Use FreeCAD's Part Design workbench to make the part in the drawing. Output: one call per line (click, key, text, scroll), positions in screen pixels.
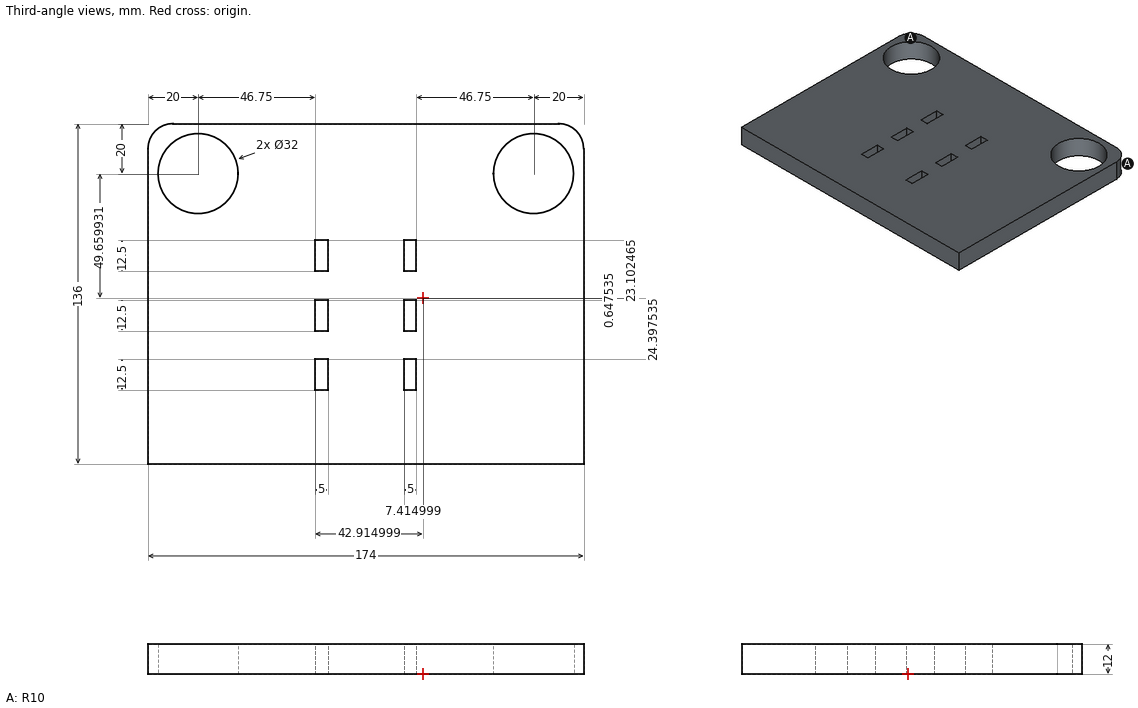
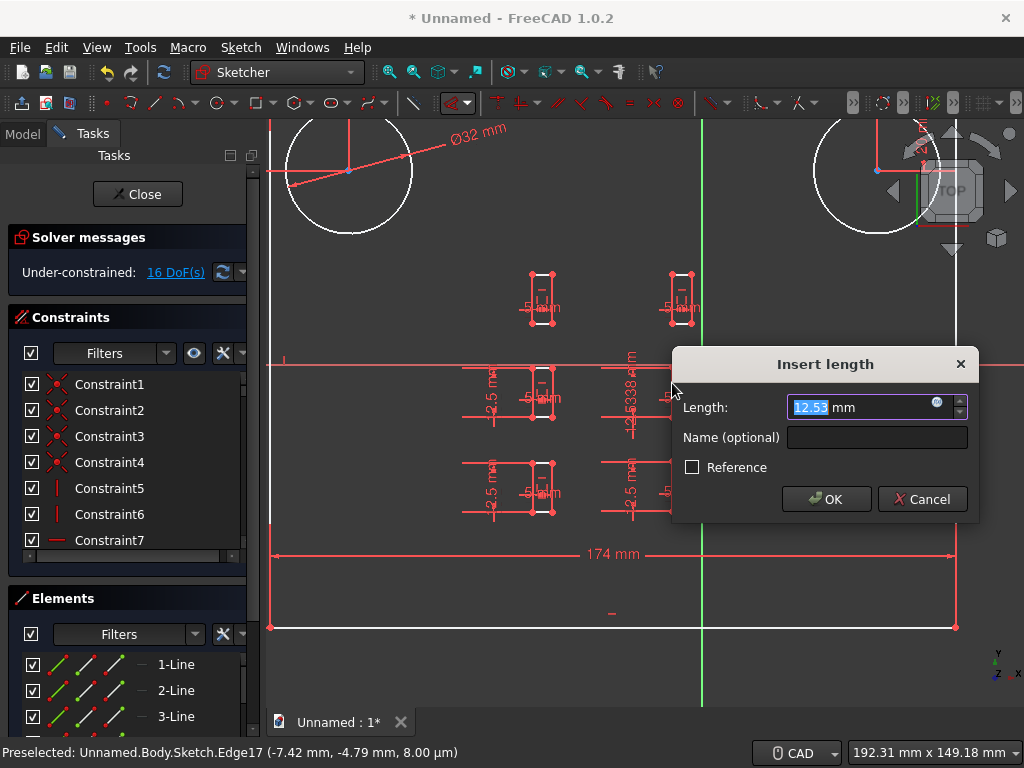
text(12.5)
key(Return)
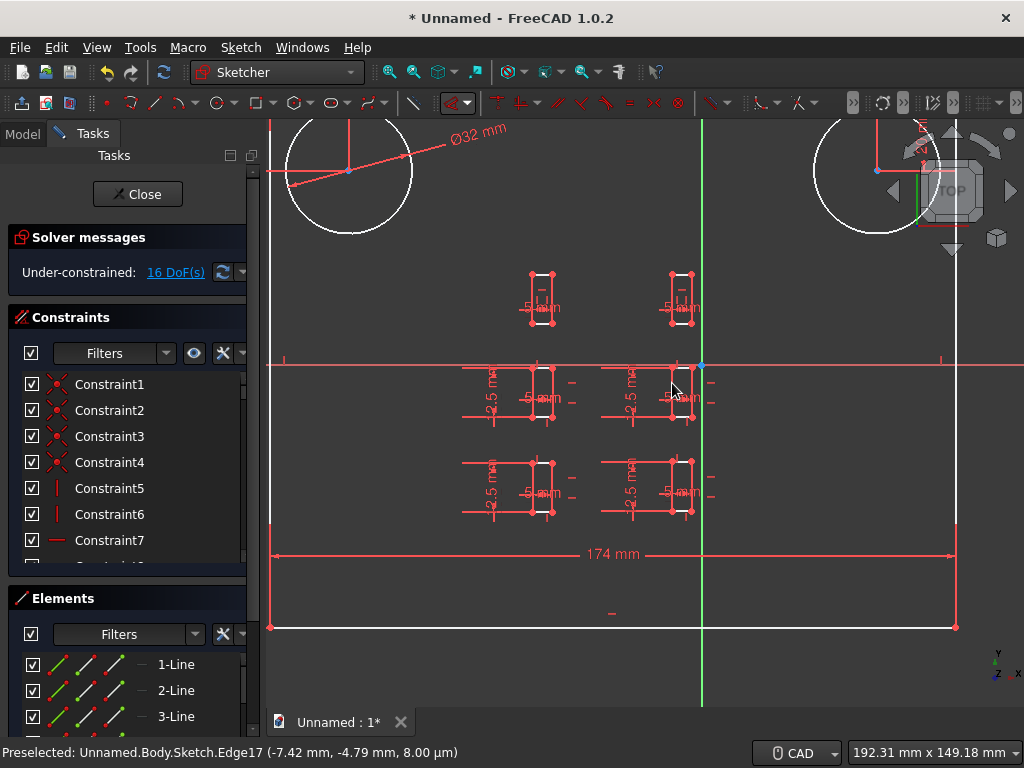
click(532, 289)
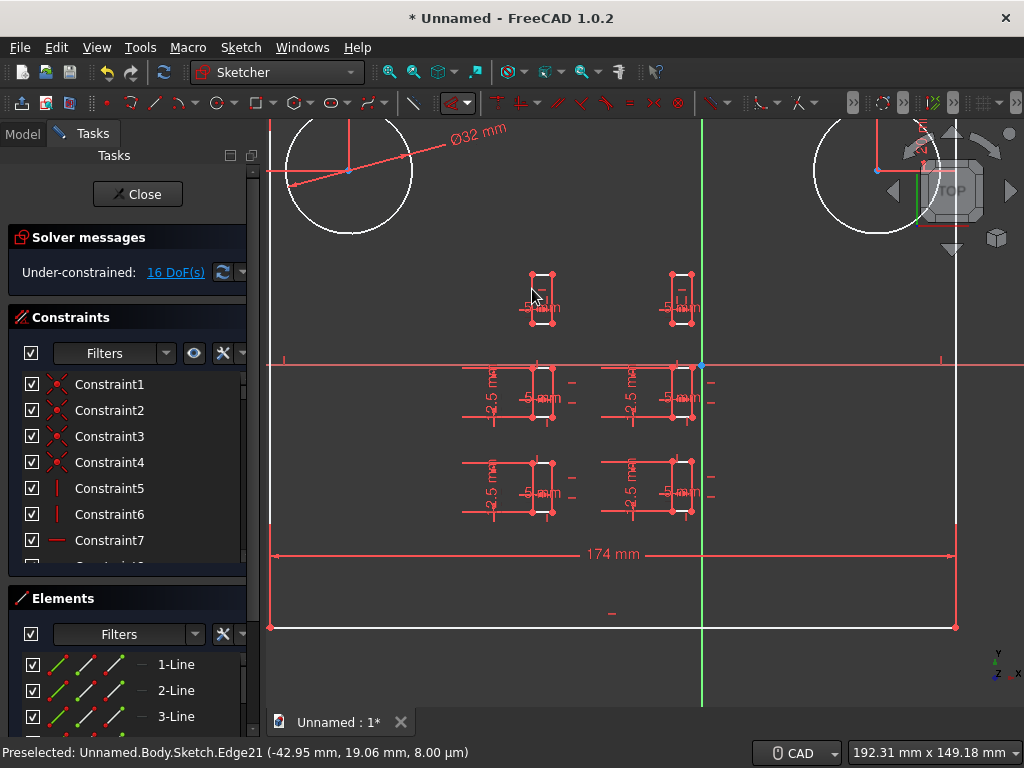
click(470, 104)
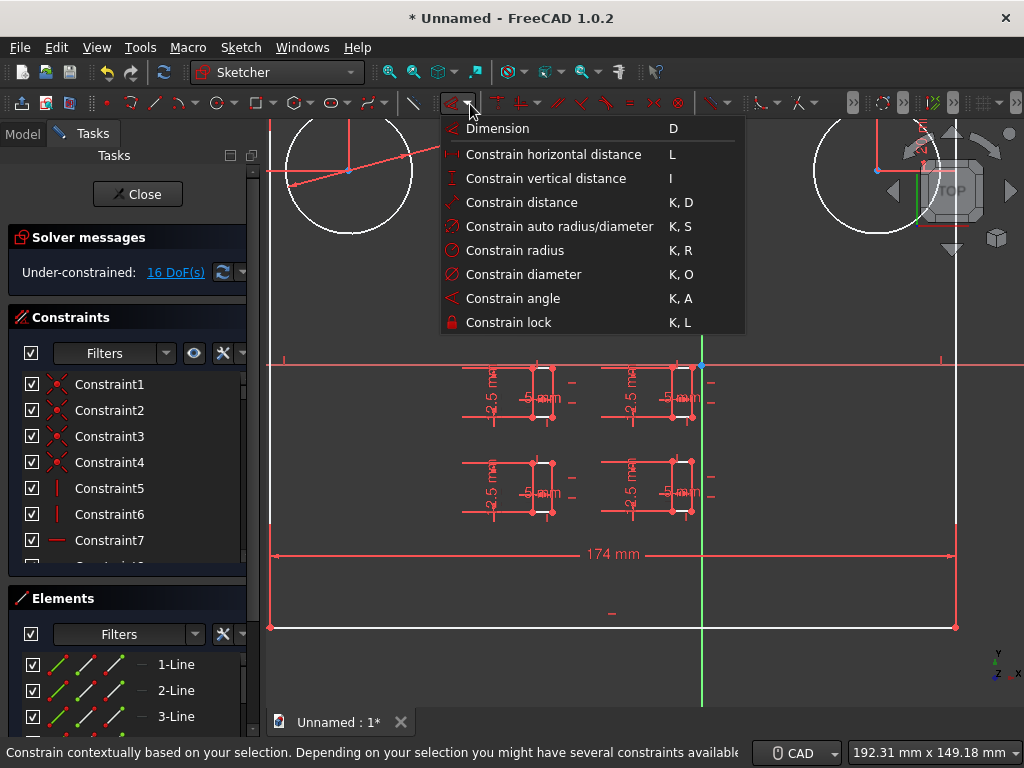
click(593, 178)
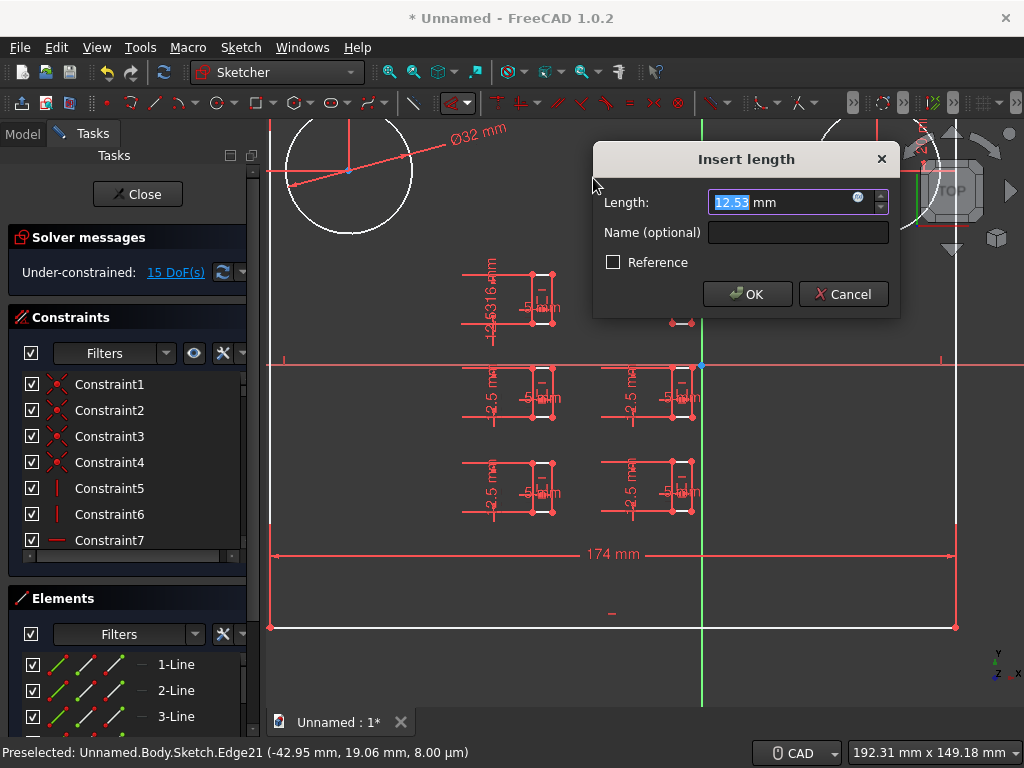
text(12.5)
key(Return)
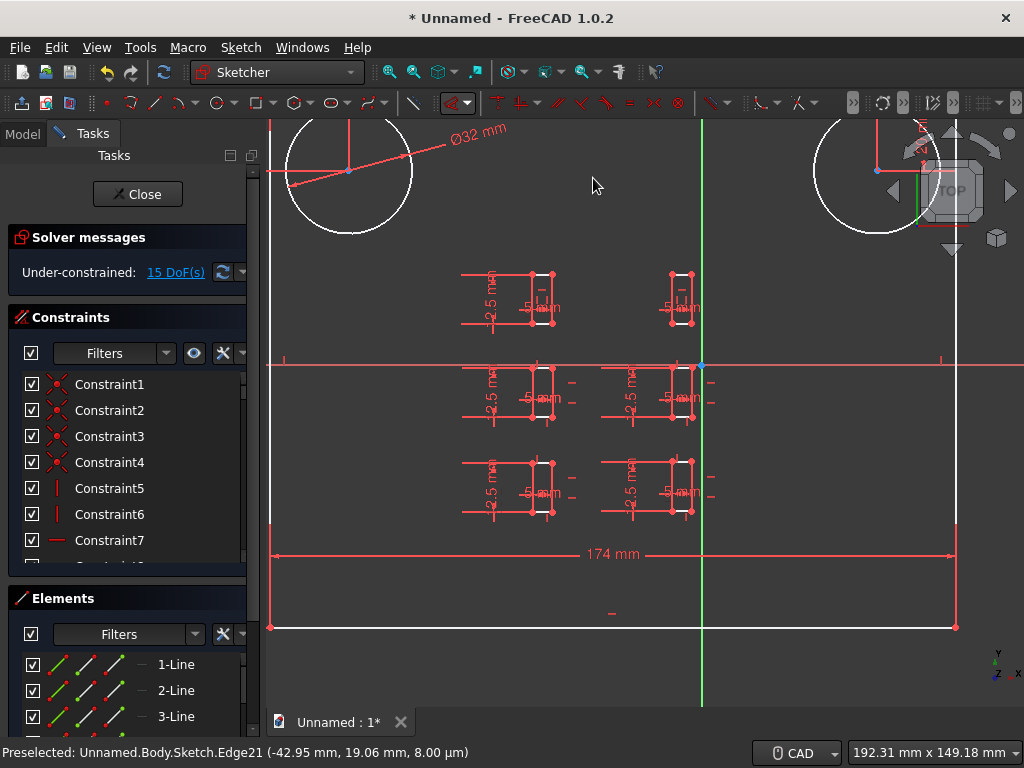
click(672, 289)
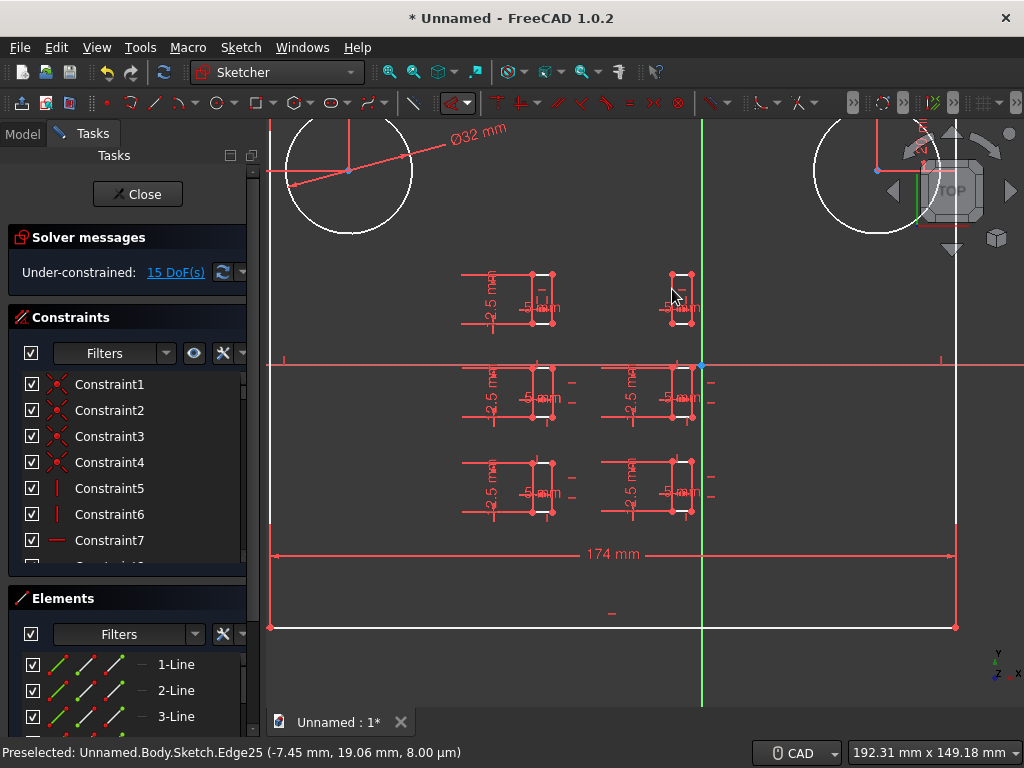
key(i)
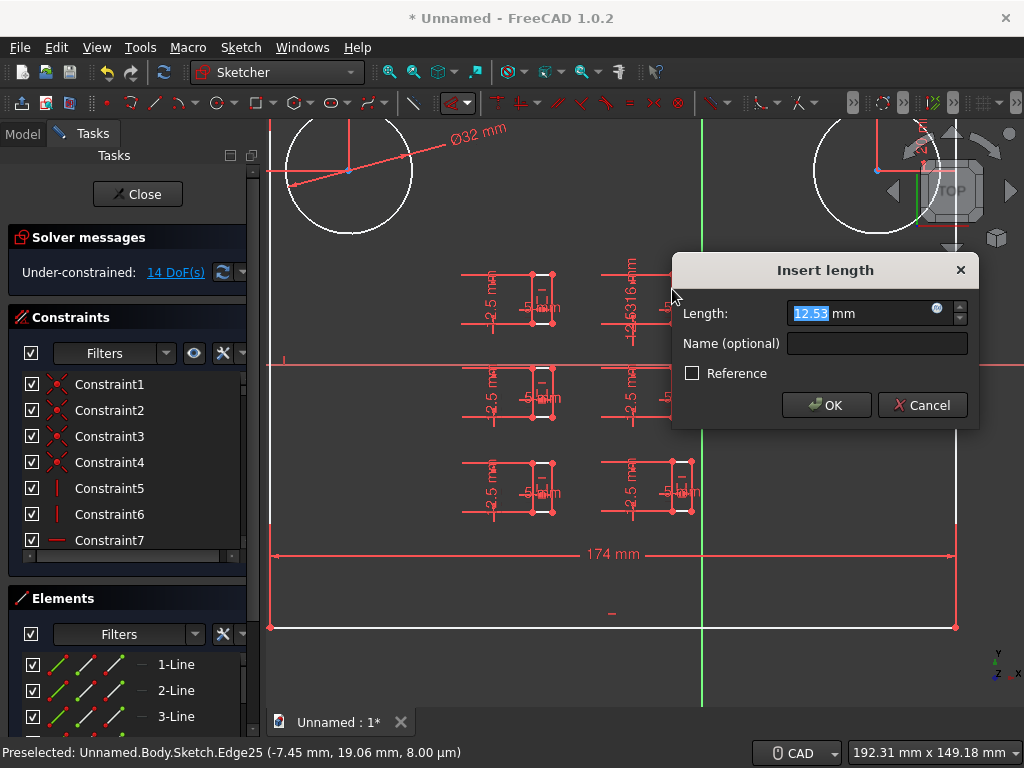
text(12.5)
key(Return)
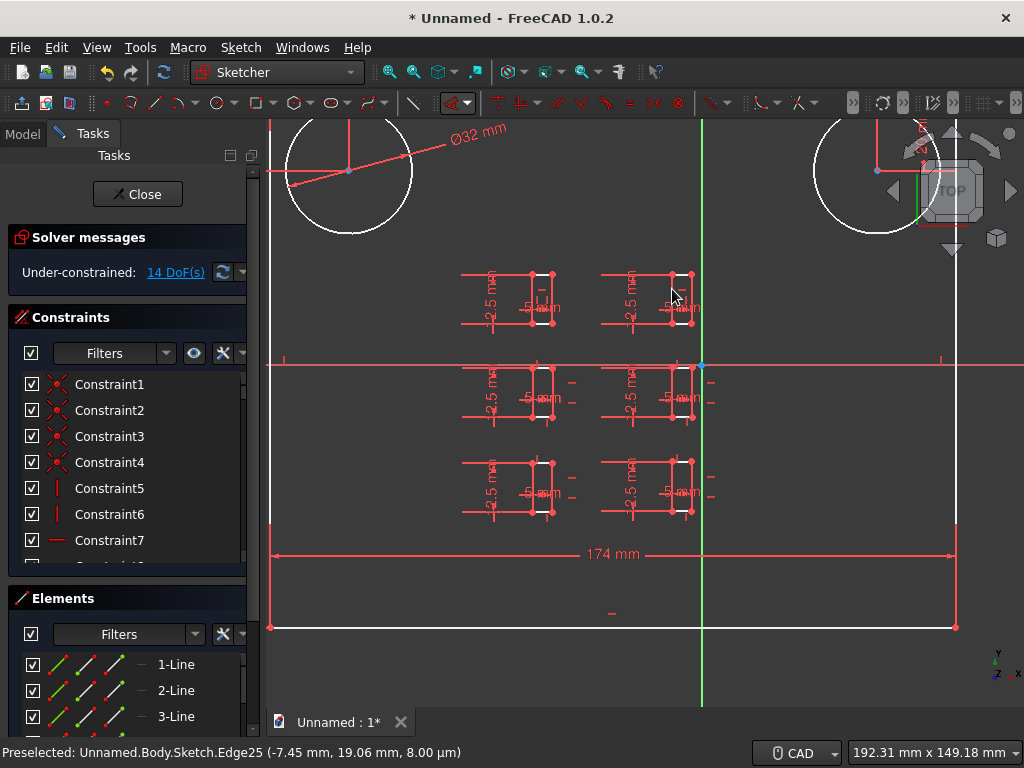
click(532, 275)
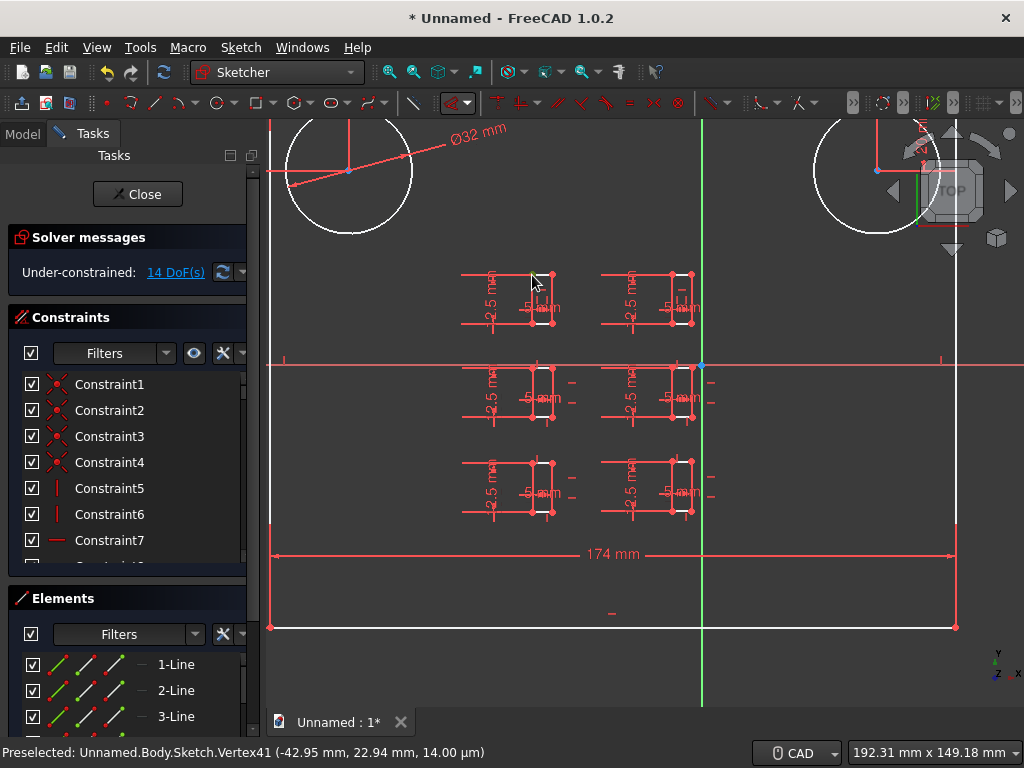
click(349, 171)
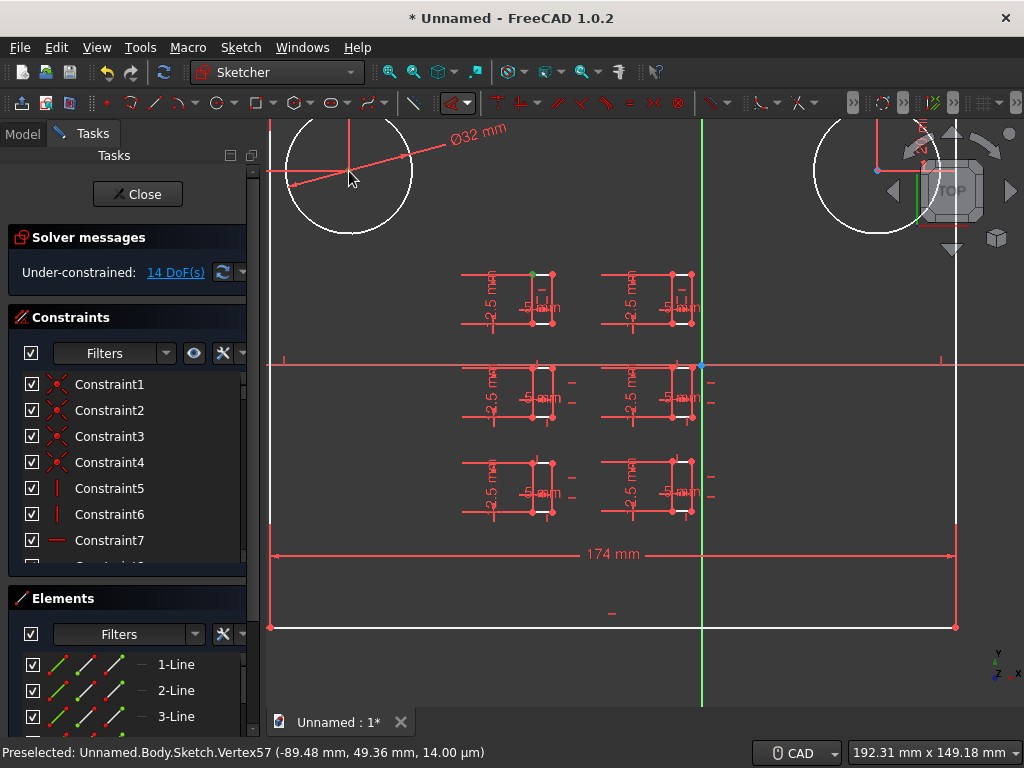
click(470, 104)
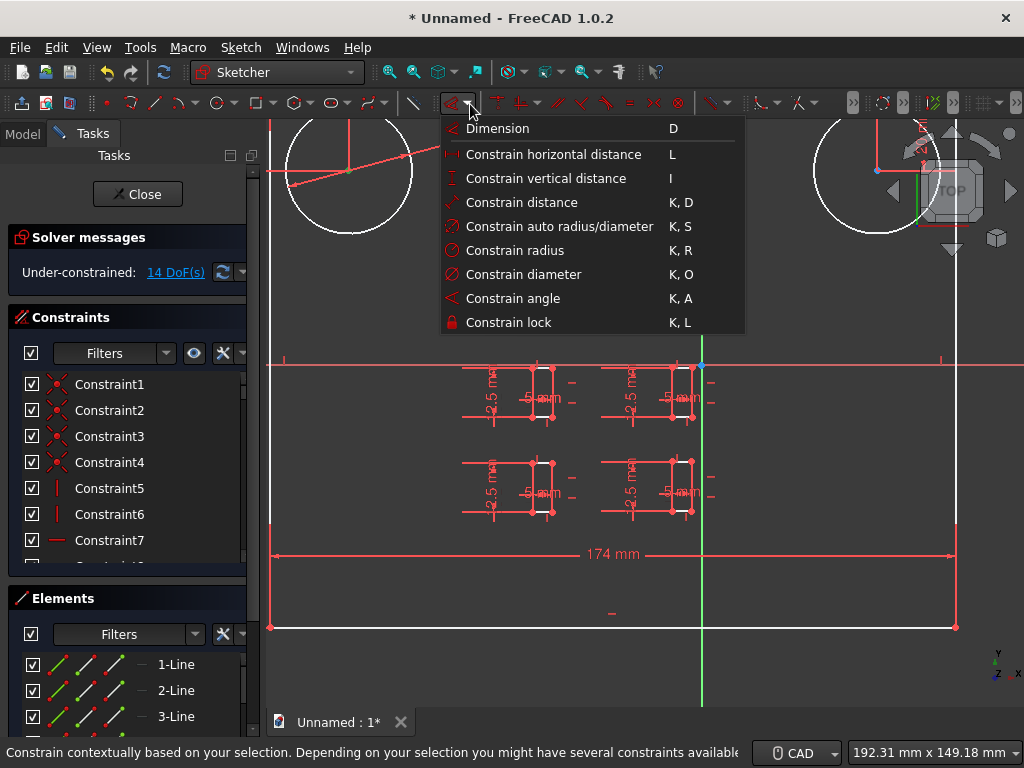
click(593, 154)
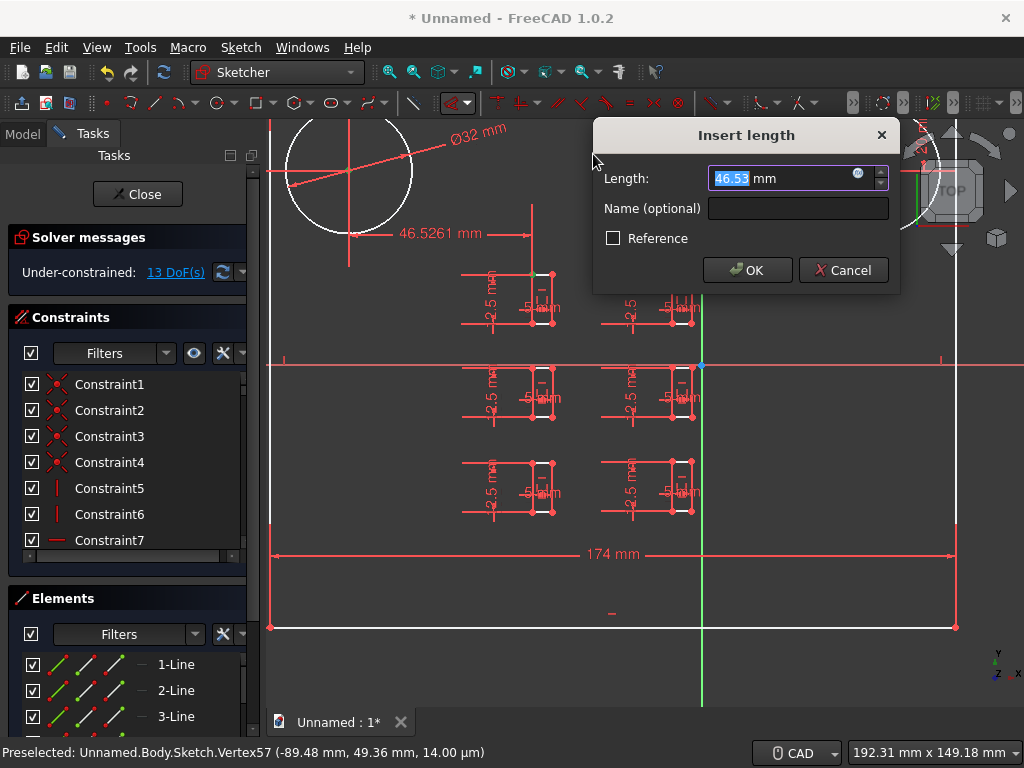
text(46.75)
key(Return)